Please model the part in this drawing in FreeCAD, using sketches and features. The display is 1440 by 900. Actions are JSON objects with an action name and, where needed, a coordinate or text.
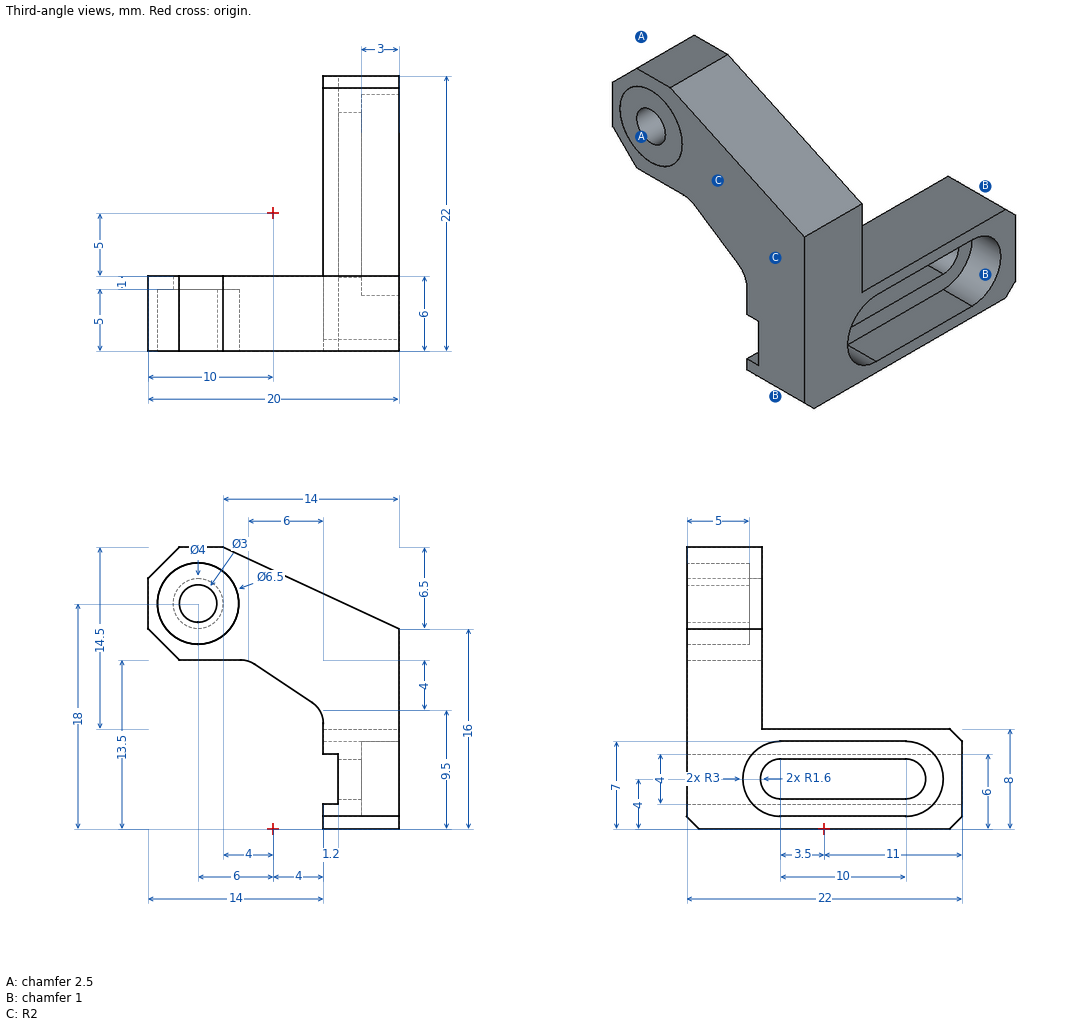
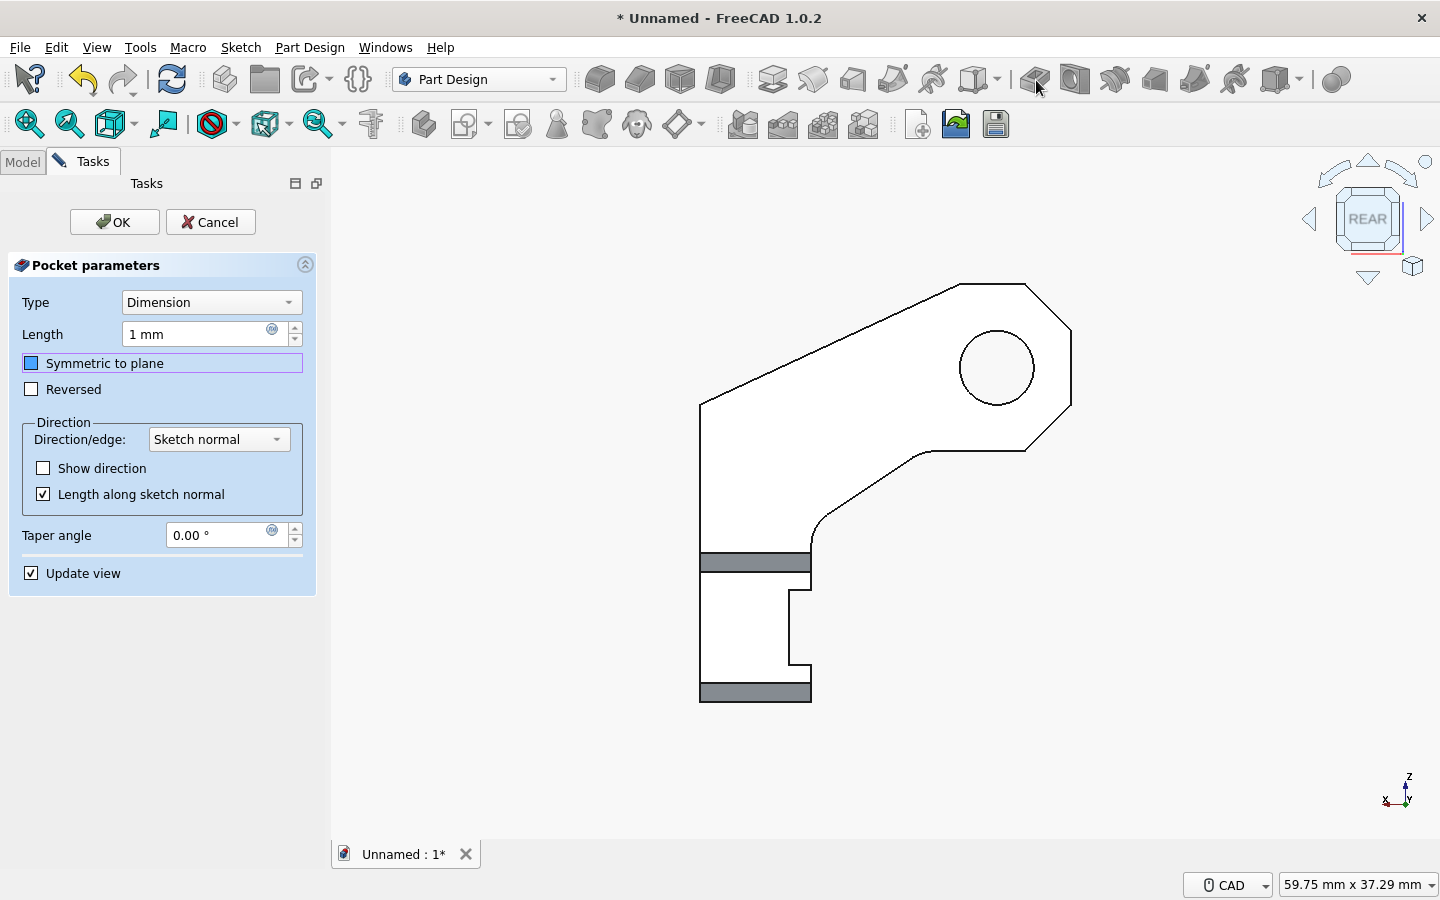
{"action": "left_click", "coordinate": [115, 222]}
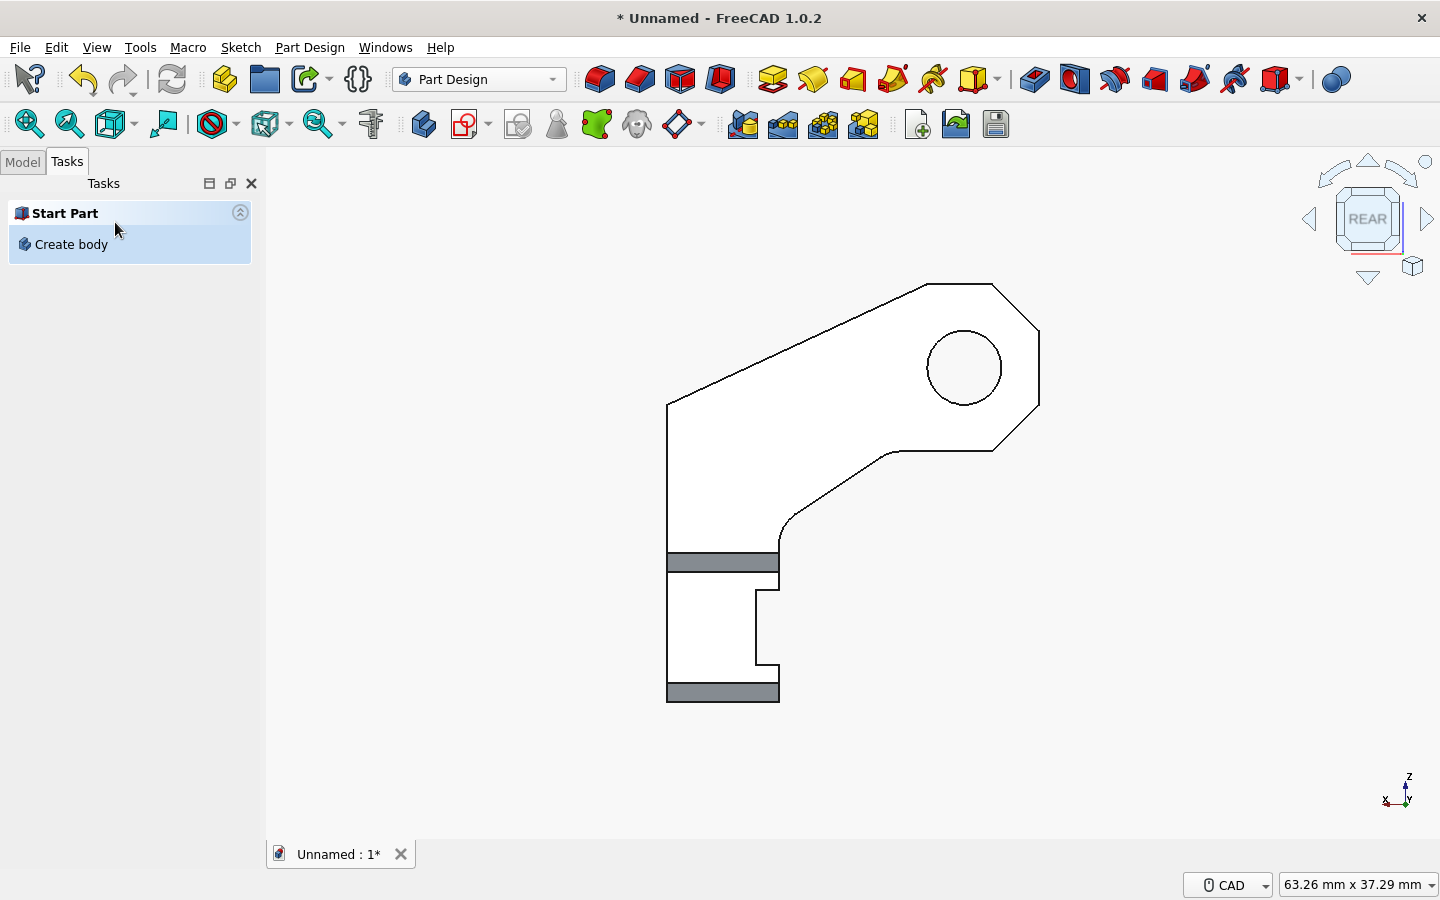
{"action": "left_click", "coordinate": [424, 124]}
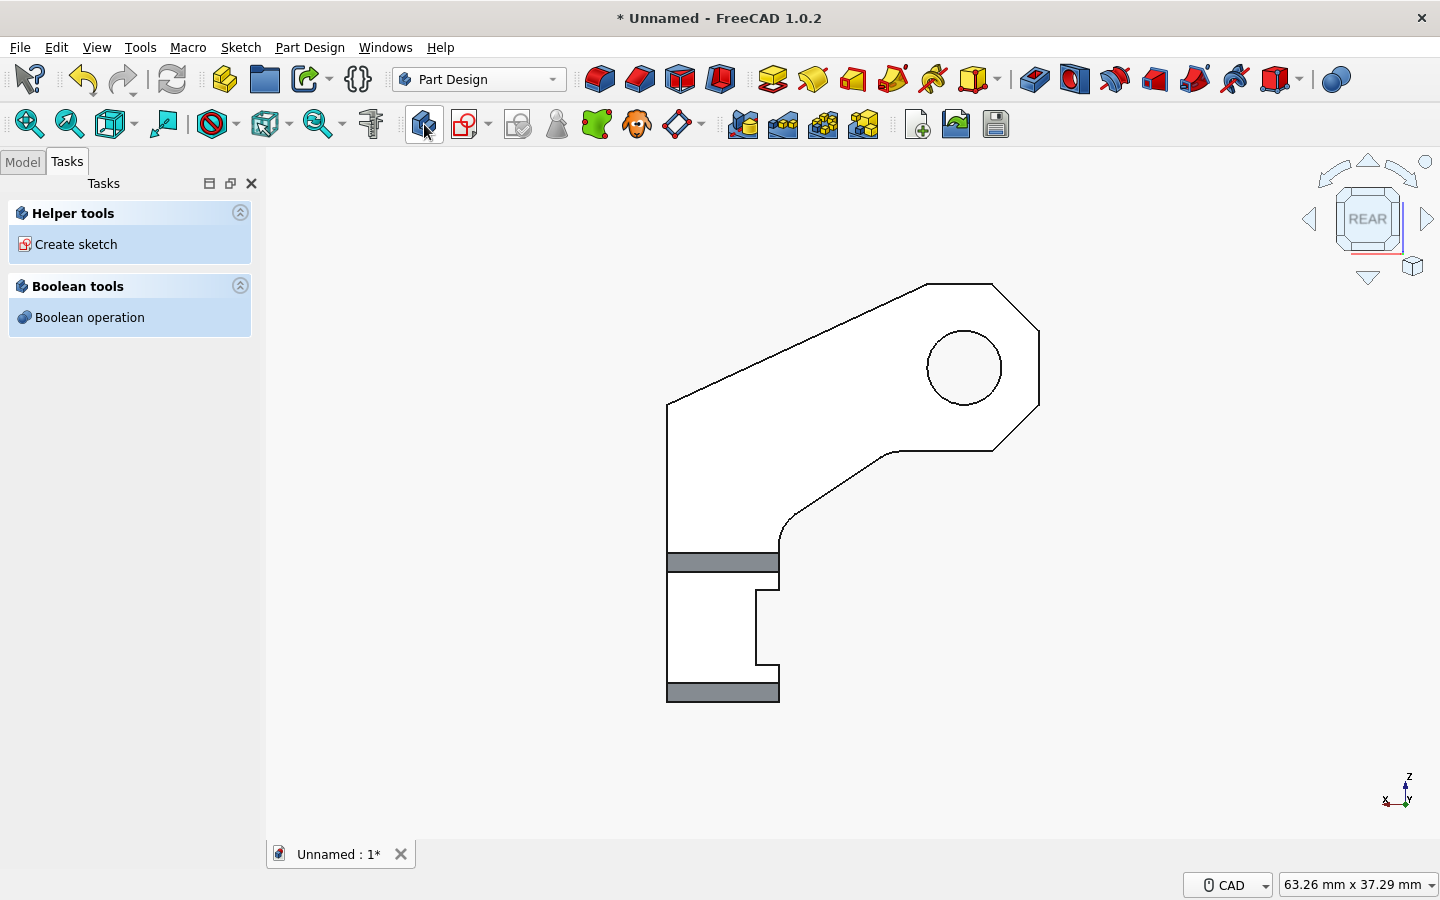
{"action": "left_click", "coordinate": [23, 161]}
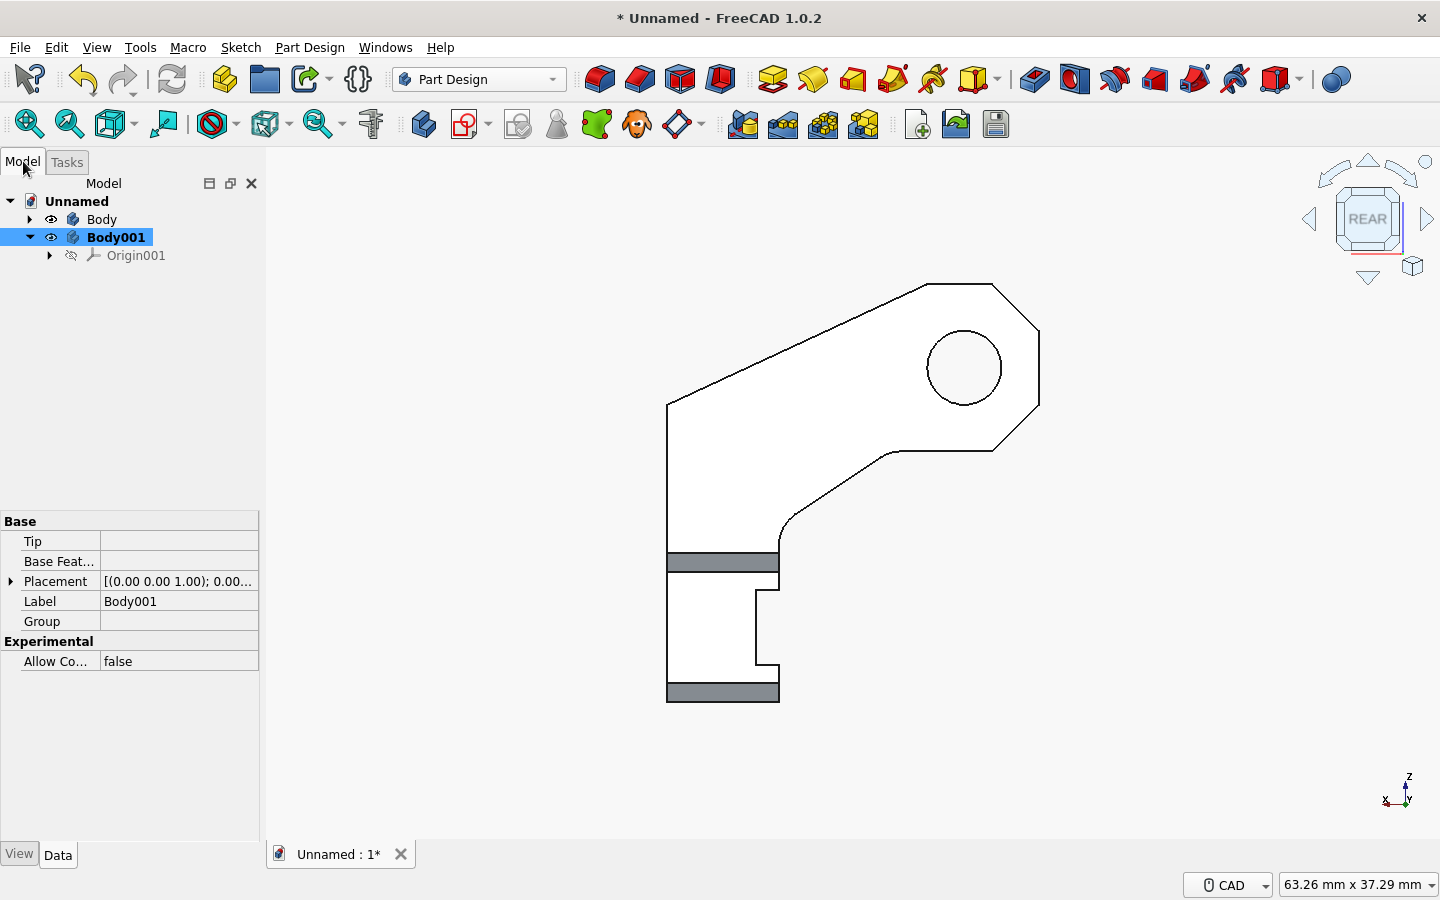
{"action": "left_click", "coordinate": [50, 255]}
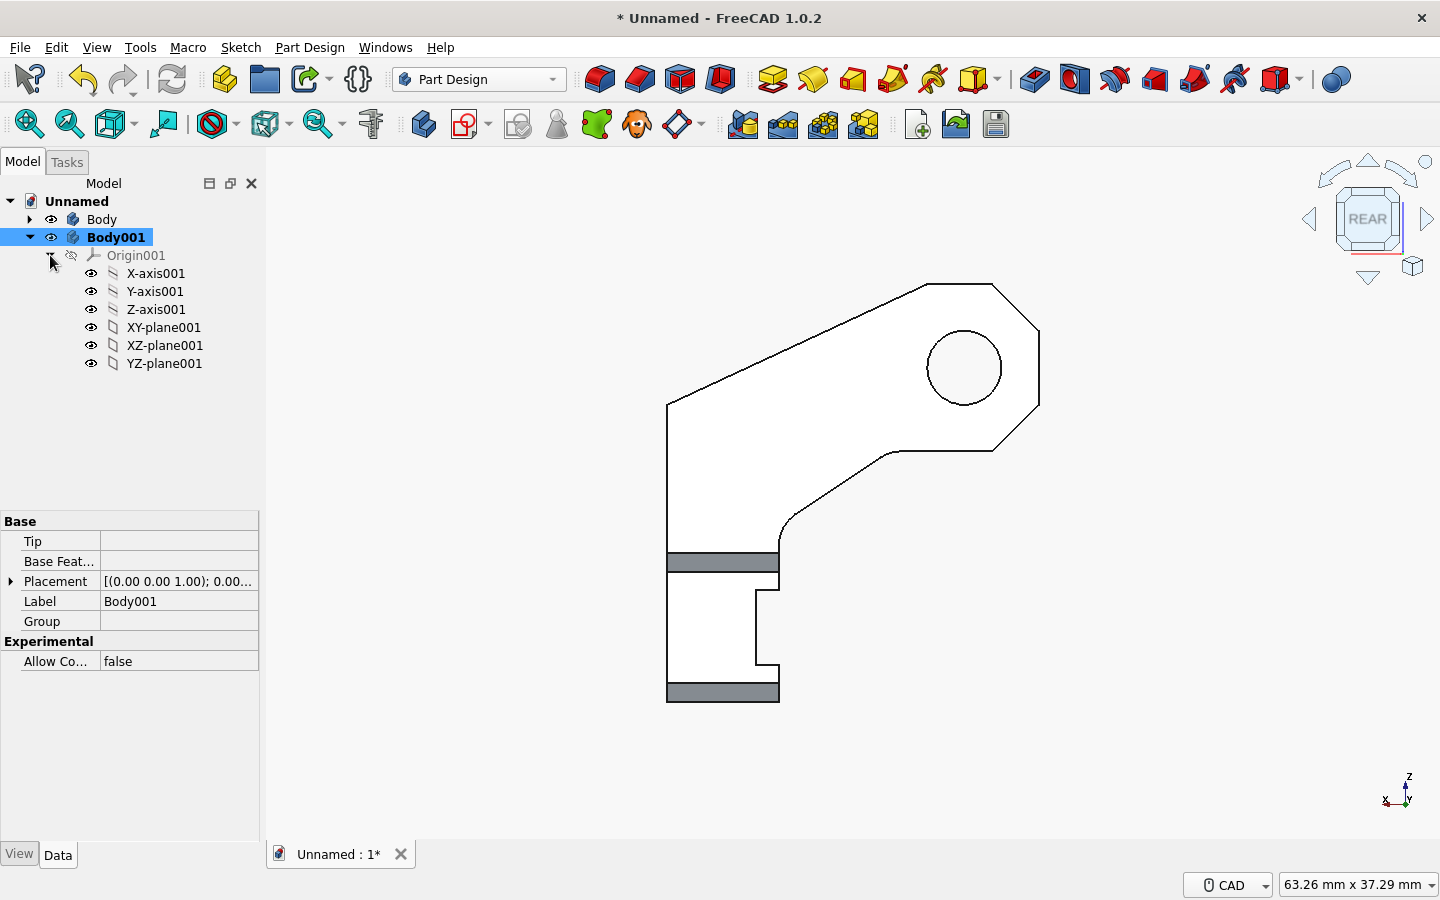
{"action": "left_click", "coordinate": [136, 345]}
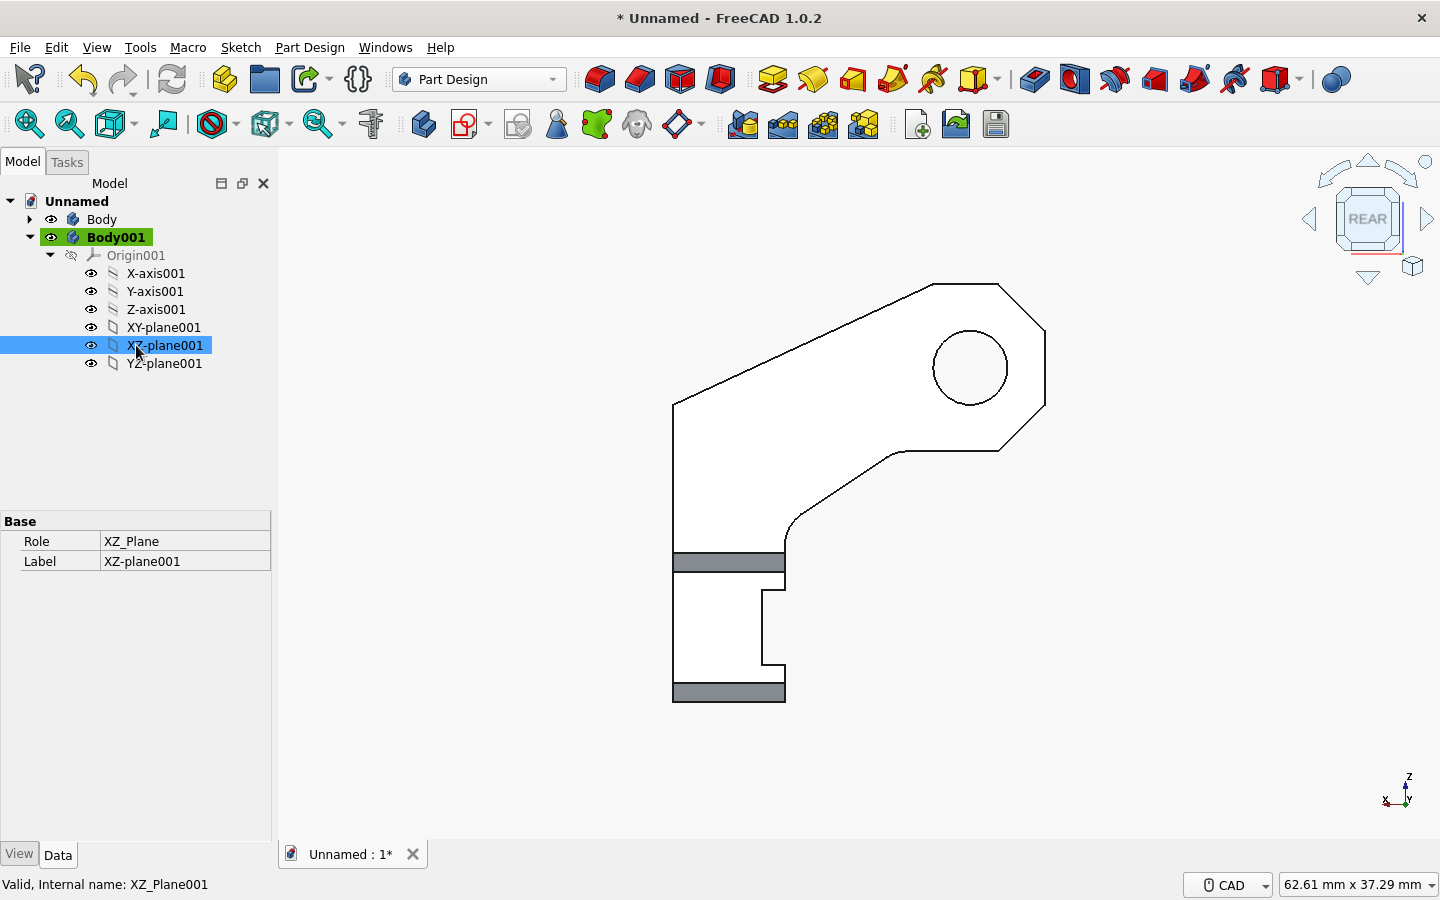
{"action": "left_click", "coordinate": [678, 124]}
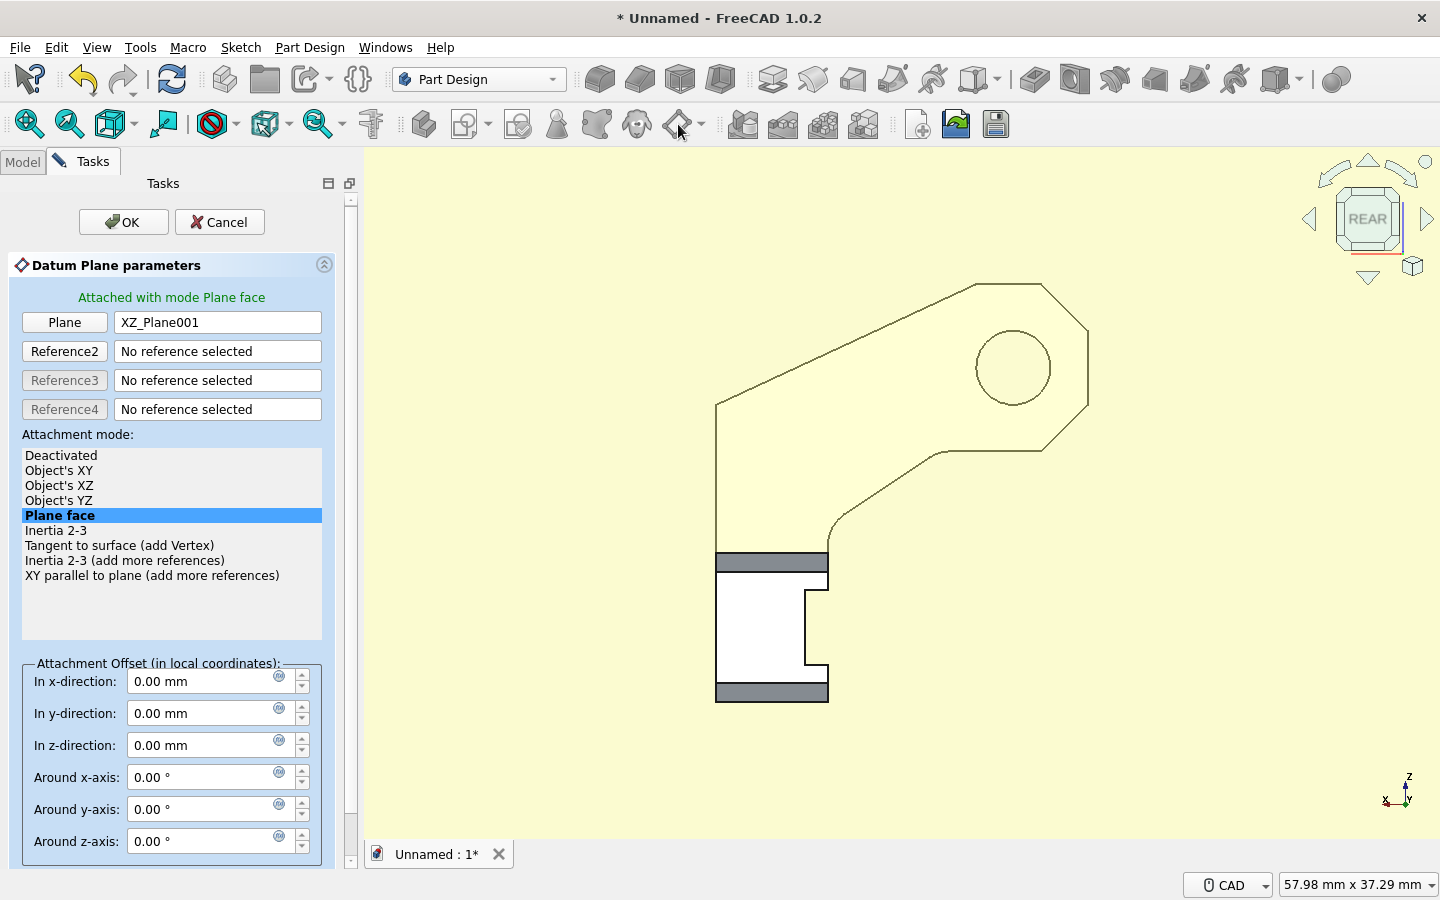
{"action": "triple_click", "coordinate": [210, 745]}